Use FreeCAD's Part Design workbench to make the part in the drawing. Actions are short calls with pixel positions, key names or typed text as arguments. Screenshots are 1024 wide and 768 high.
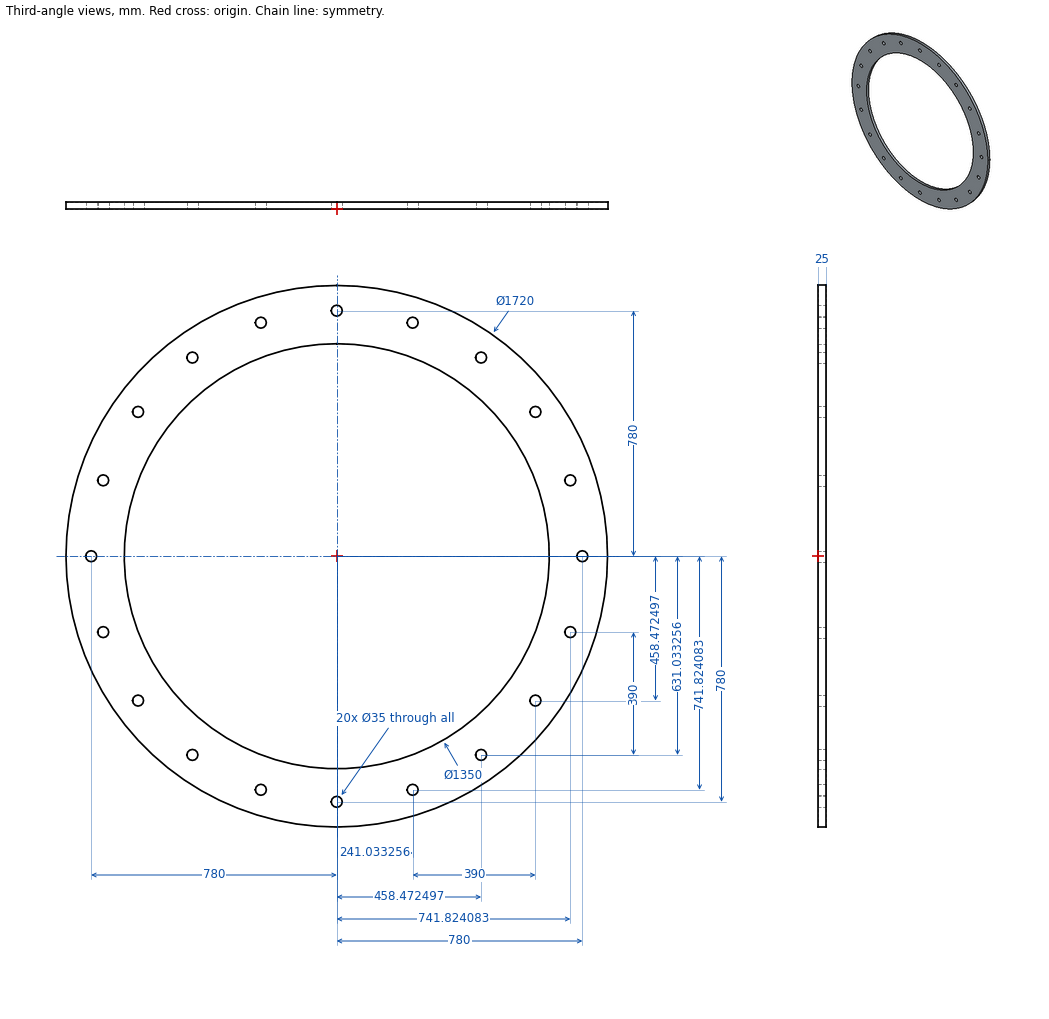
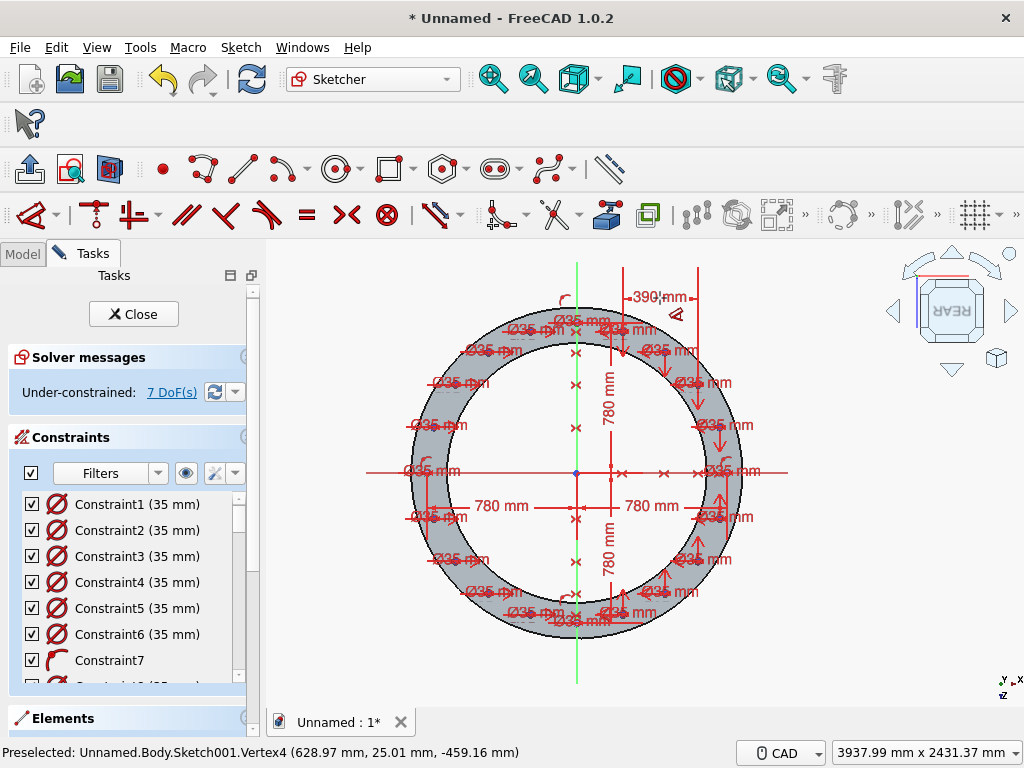
click(665, 352)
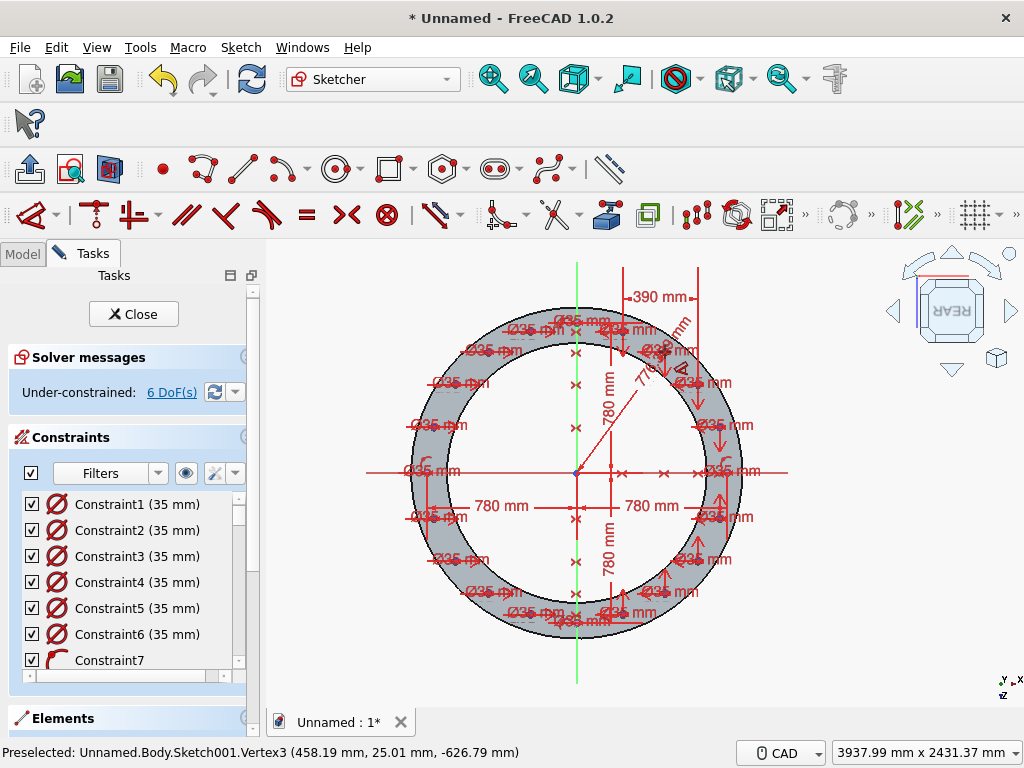
click(720, 427)
click(754, 390)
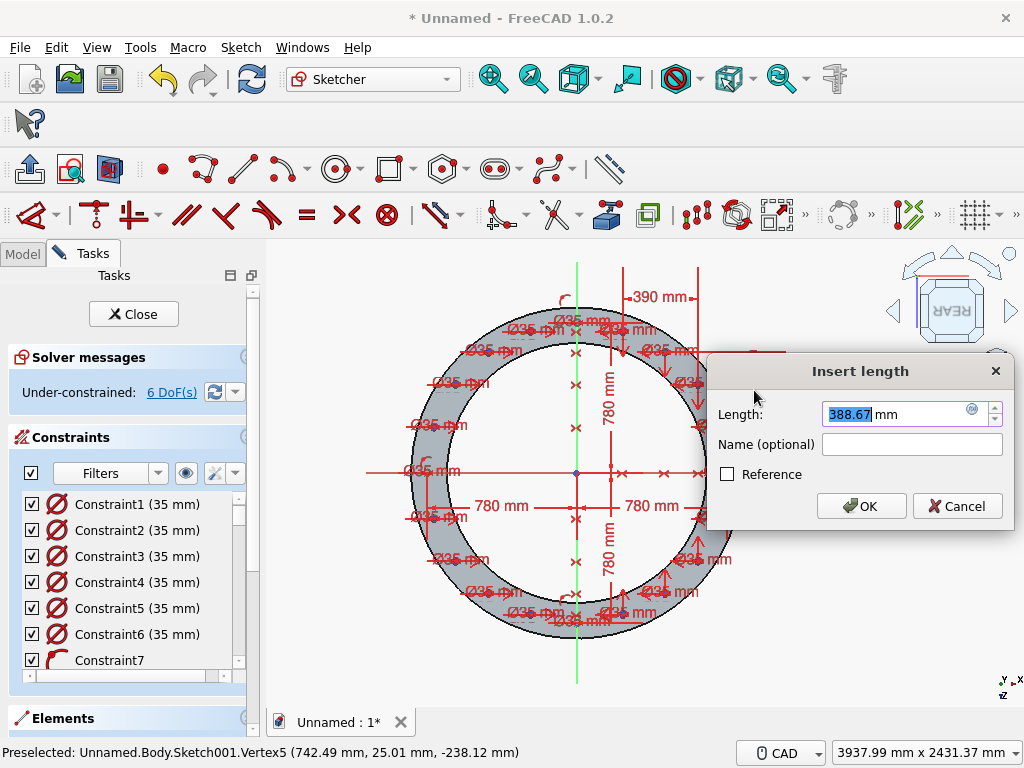
text(390)
key(Return)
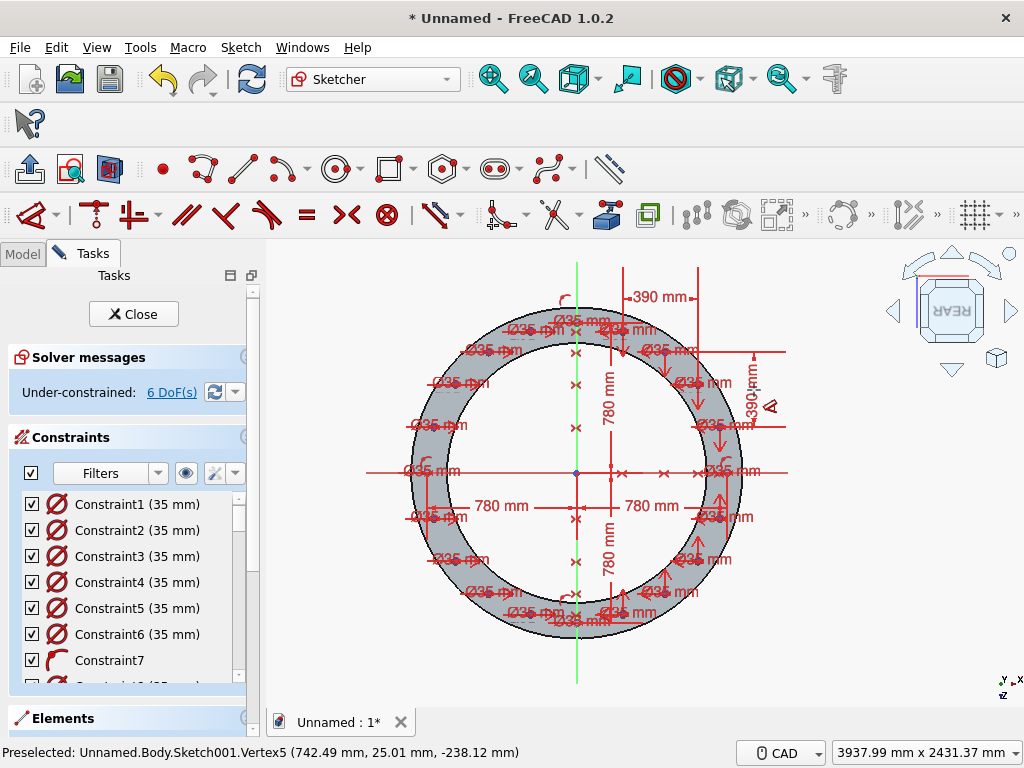
click(623, 332)
click(600, 274)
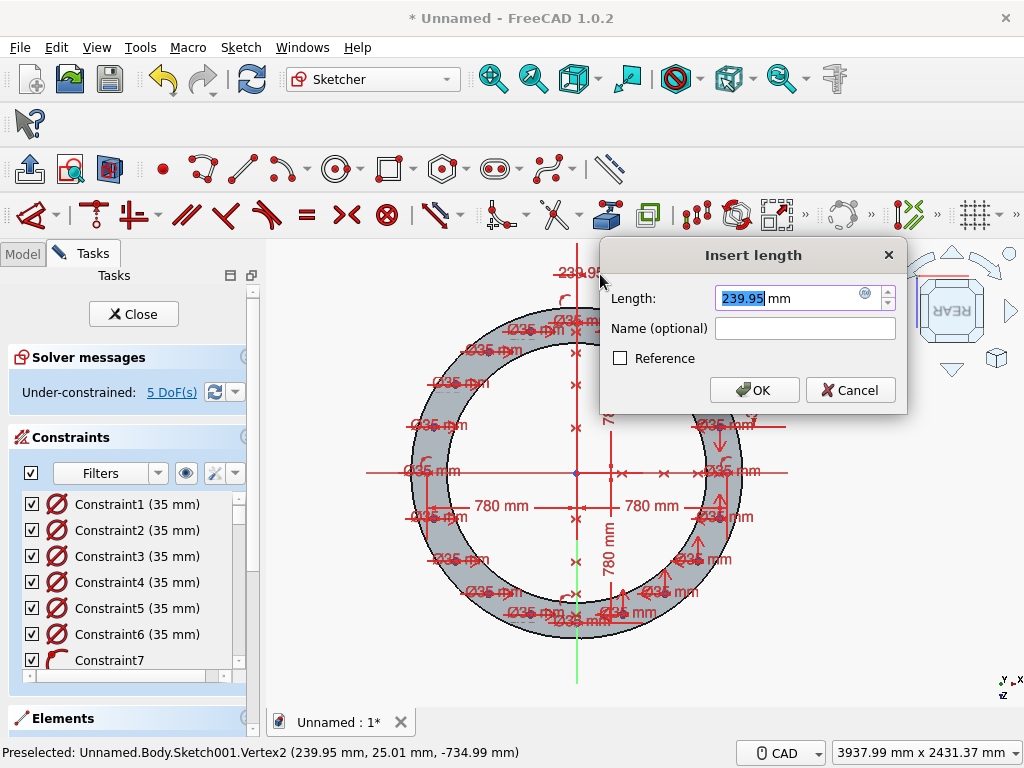
text(241.033256)
key(Return)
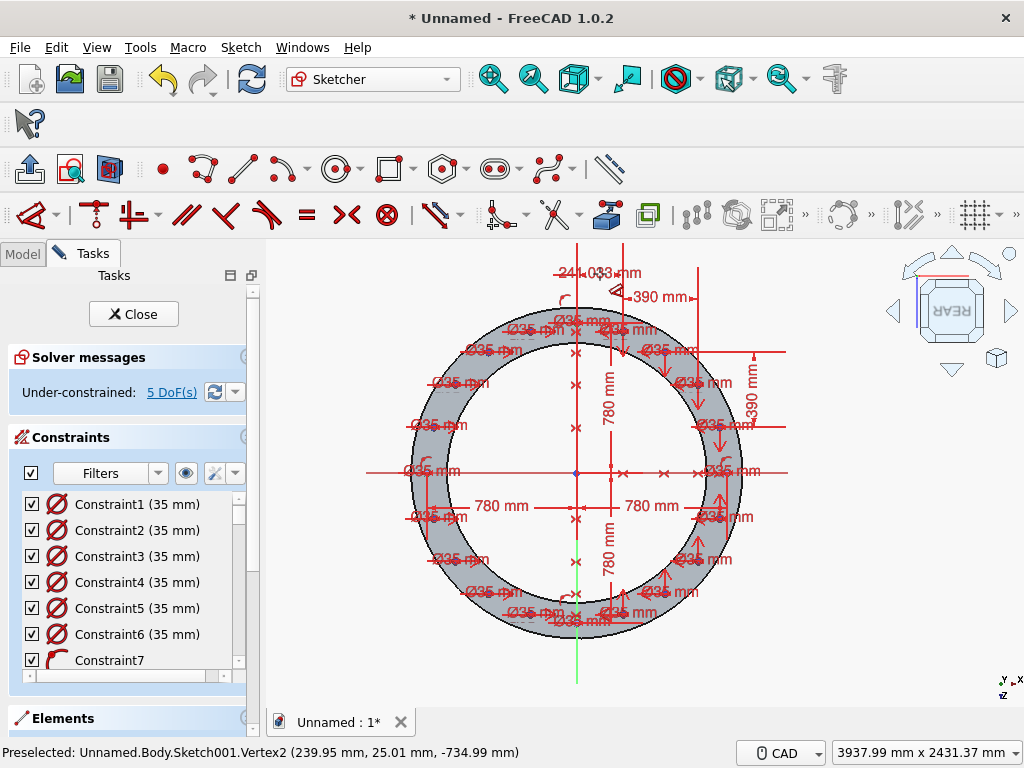
click(623, 332)
click(657, 370)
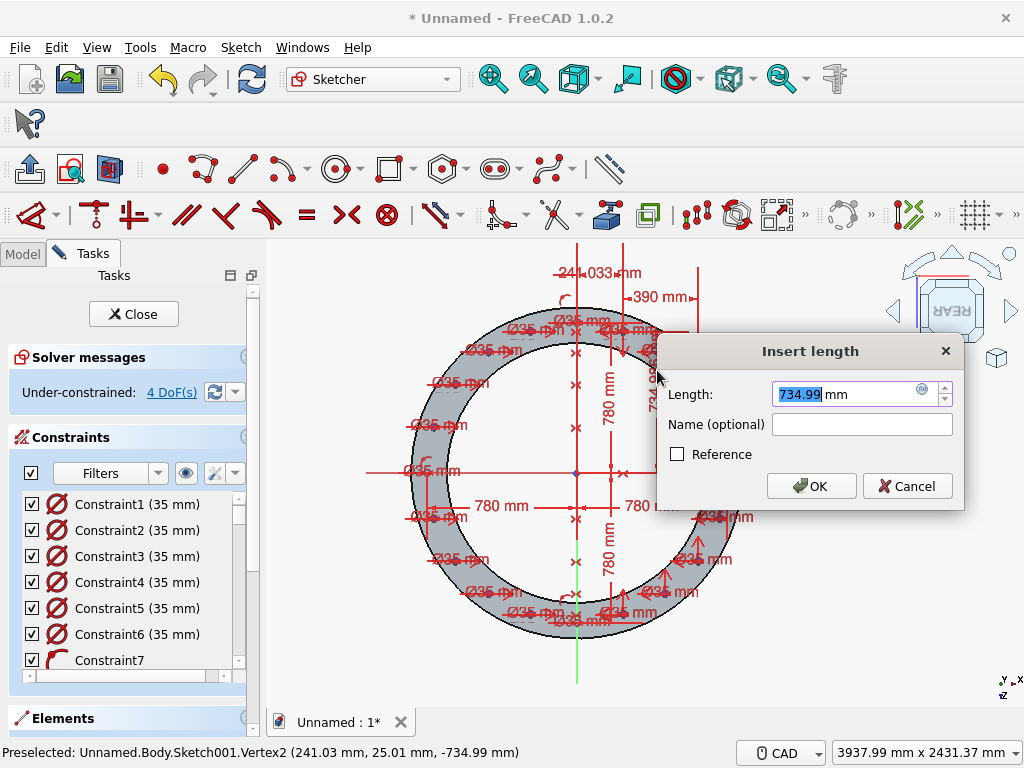
text(741.824083)
key(Return)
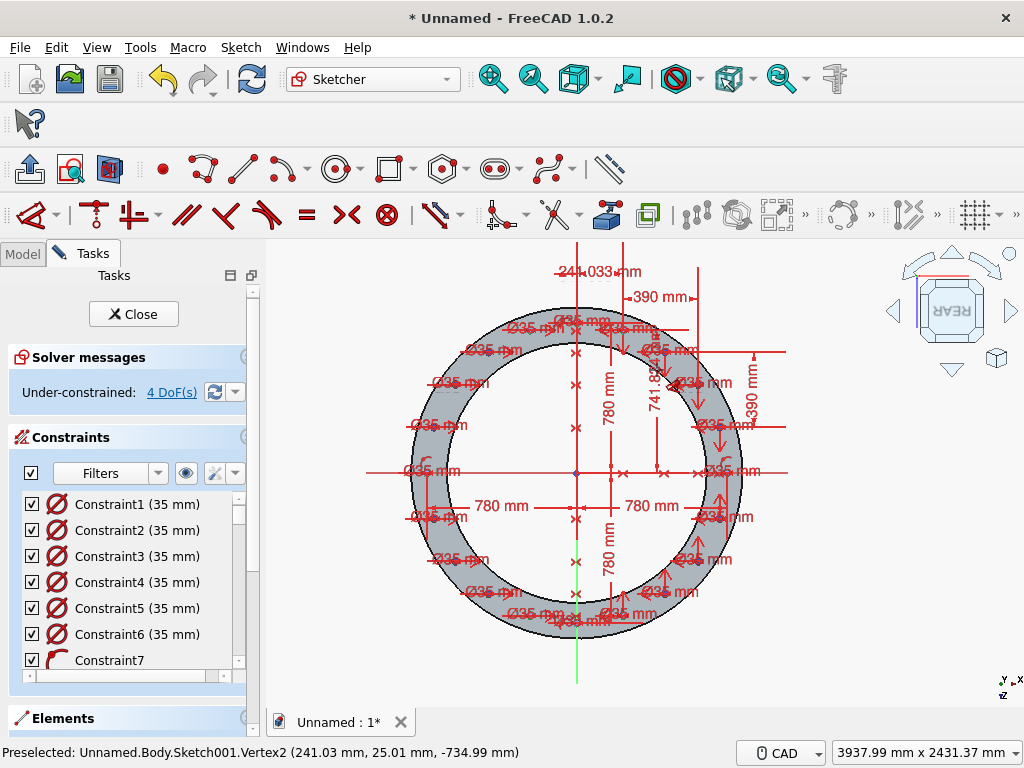
click(665, 352)
click(601, 318)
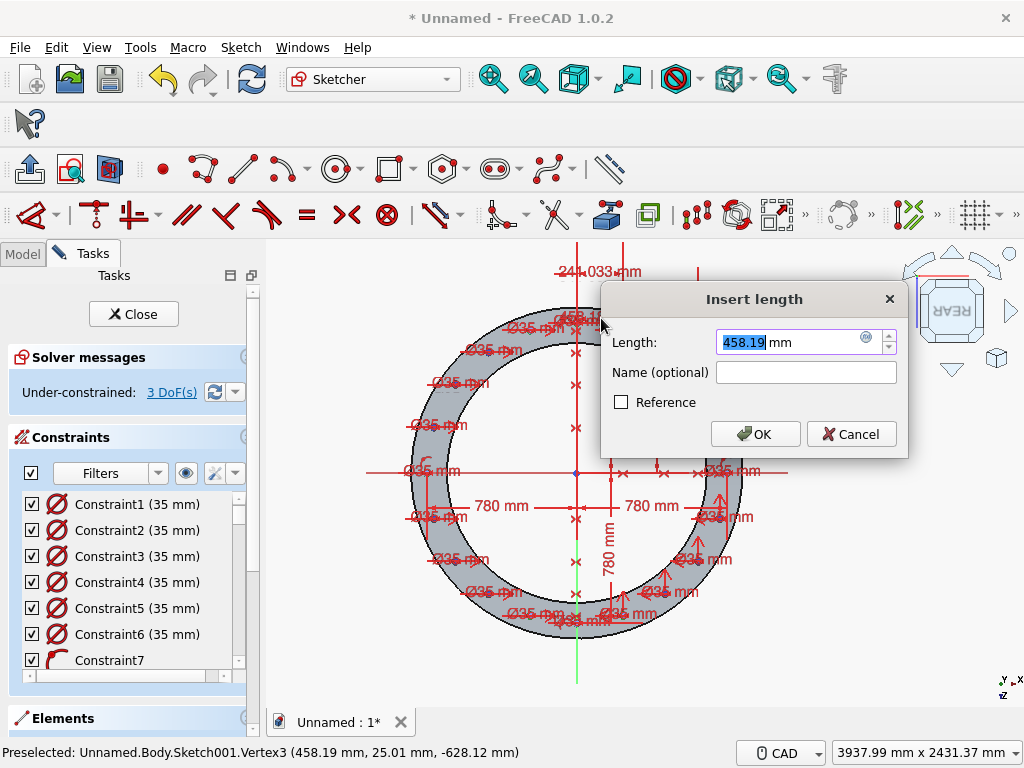
text(458.472497)
key(Return)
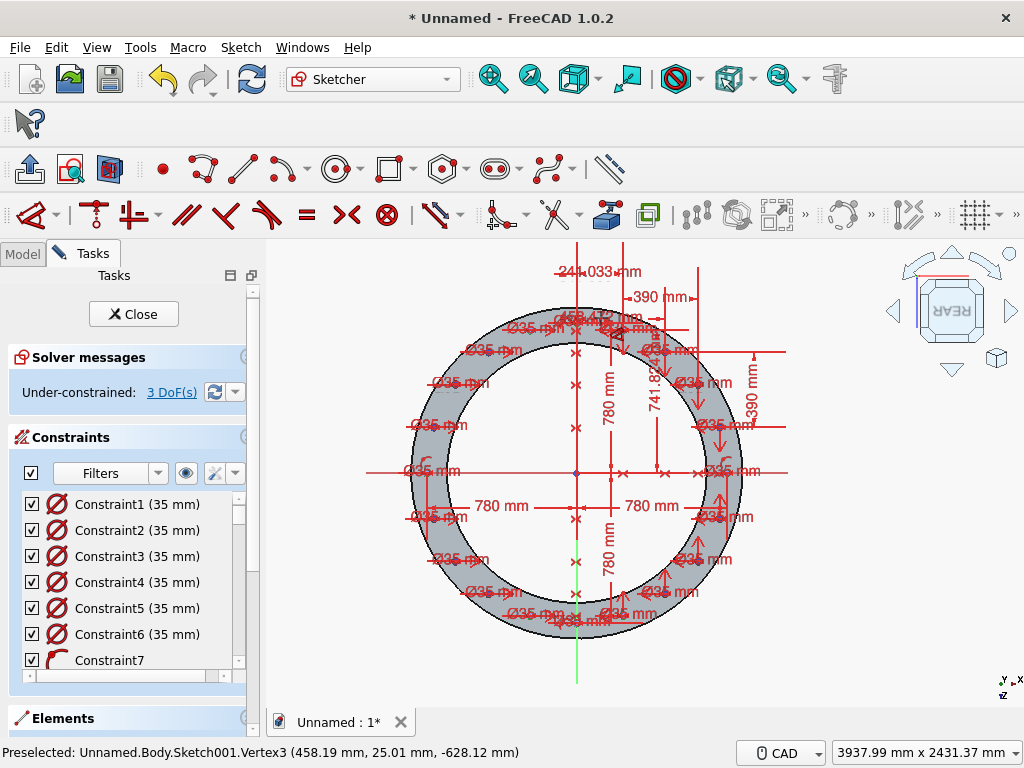
click(665, 352)
click(699, 413)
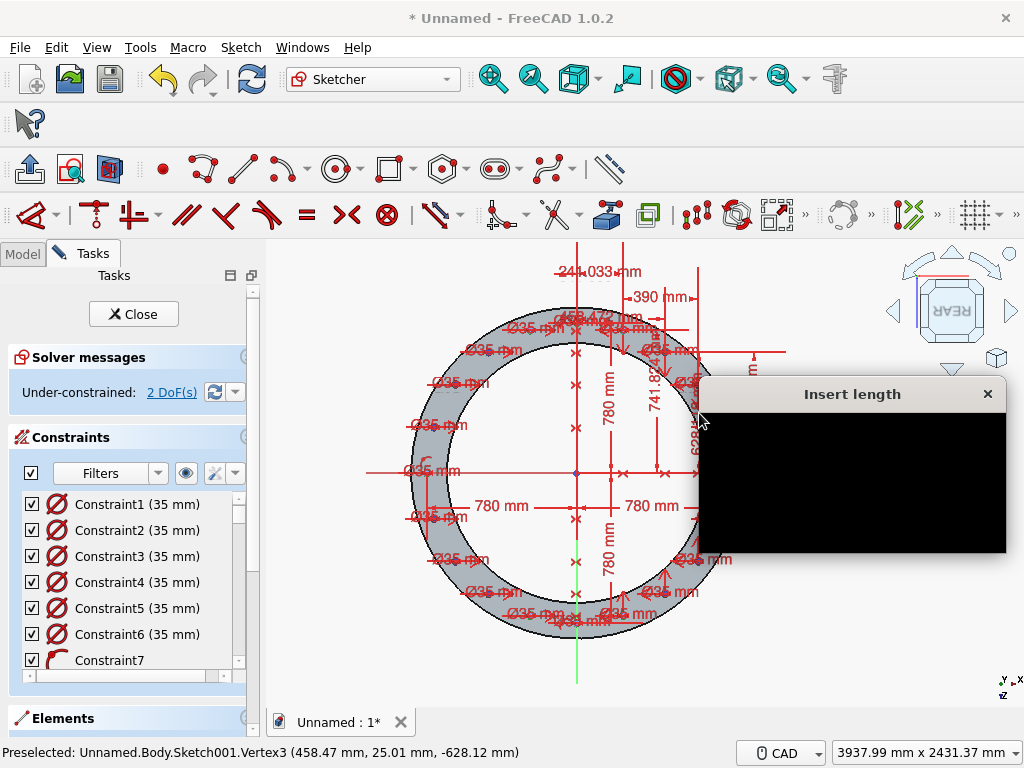
text(631.033256)
key(Return)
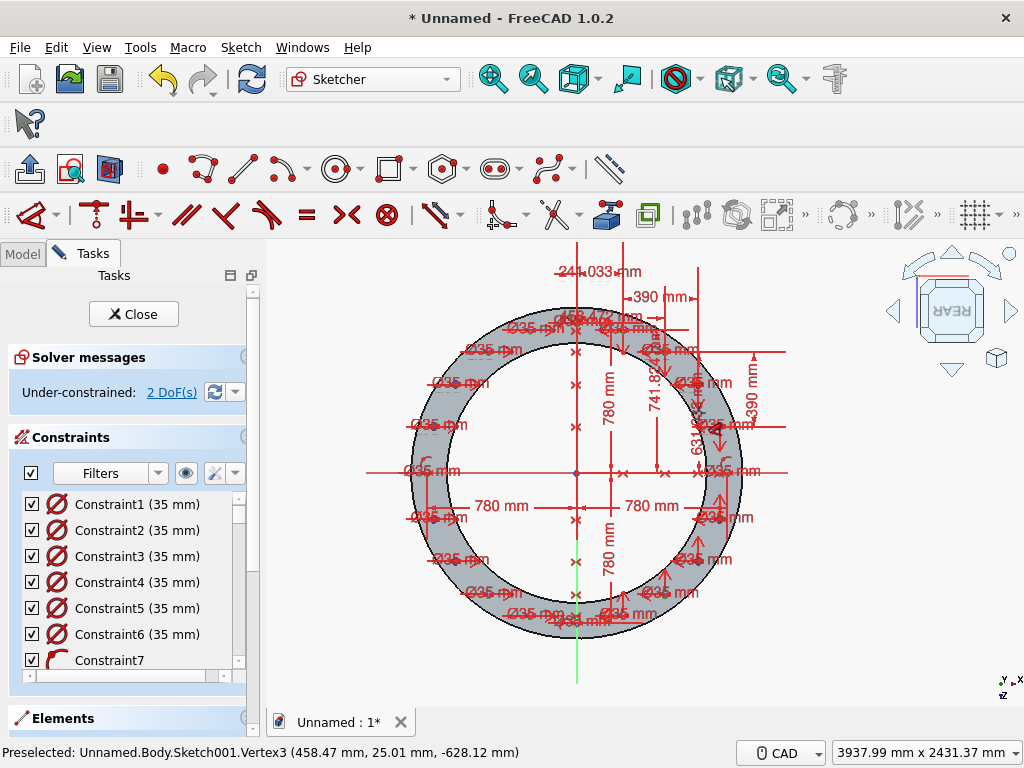
click(698, 385)
click(732, 449)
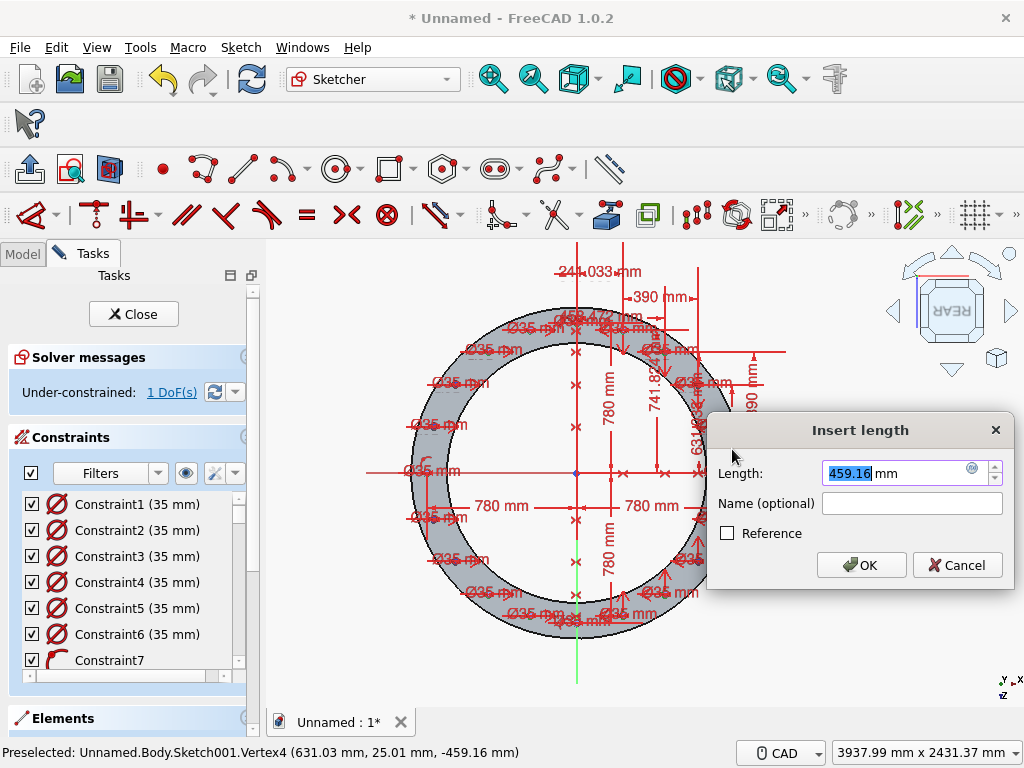
text(458.472497)
key(Return)